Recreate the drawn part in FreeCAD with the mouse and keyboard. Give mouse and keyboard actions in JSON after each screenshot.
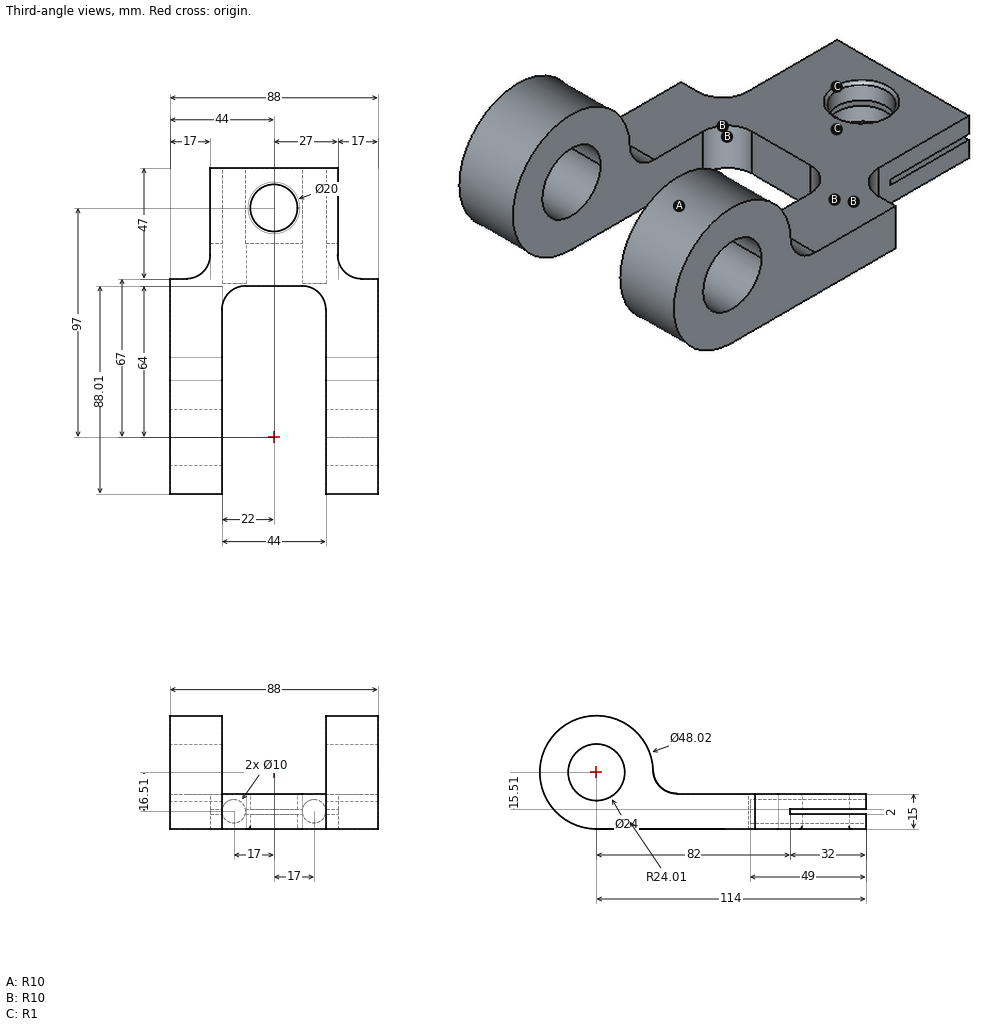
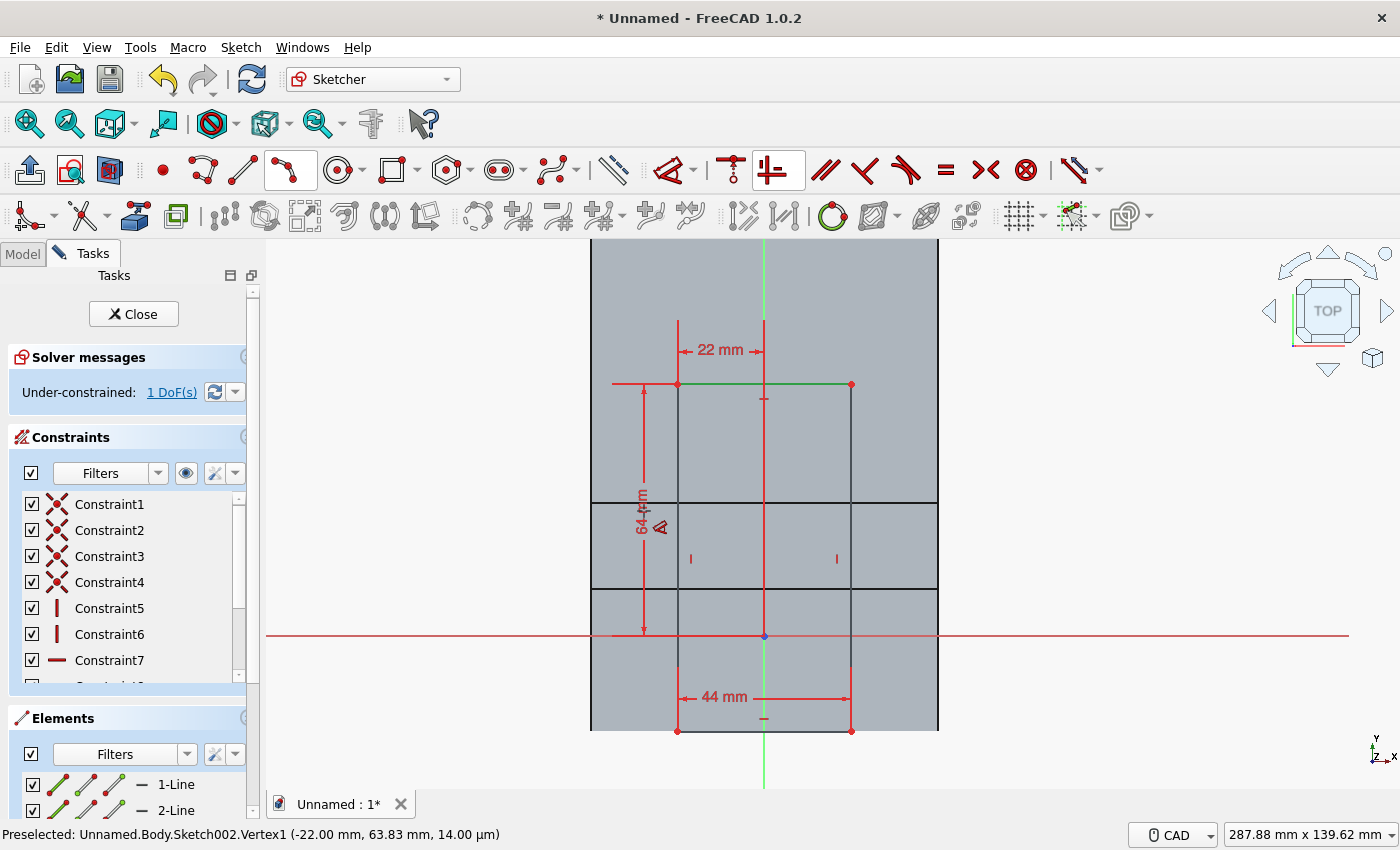
{"action": "left_click", "coordinate": [678, 489]}
{"action": "left_click", "coordinate": [644, 558]}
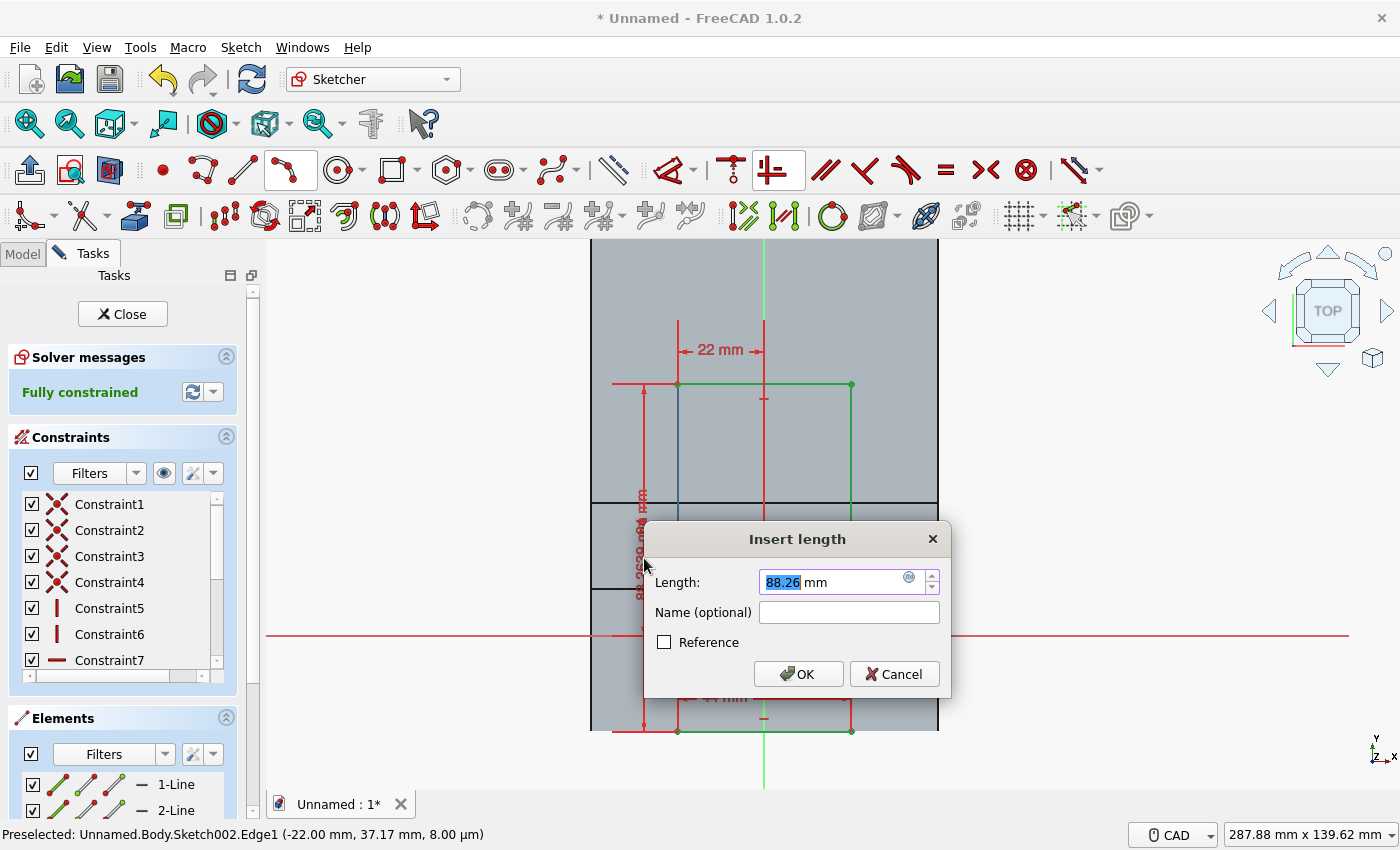
{"action": "type", "text": "88.01"}
{"action": "key", "text": "Return"}
{"action": "key", "text": "Escape"}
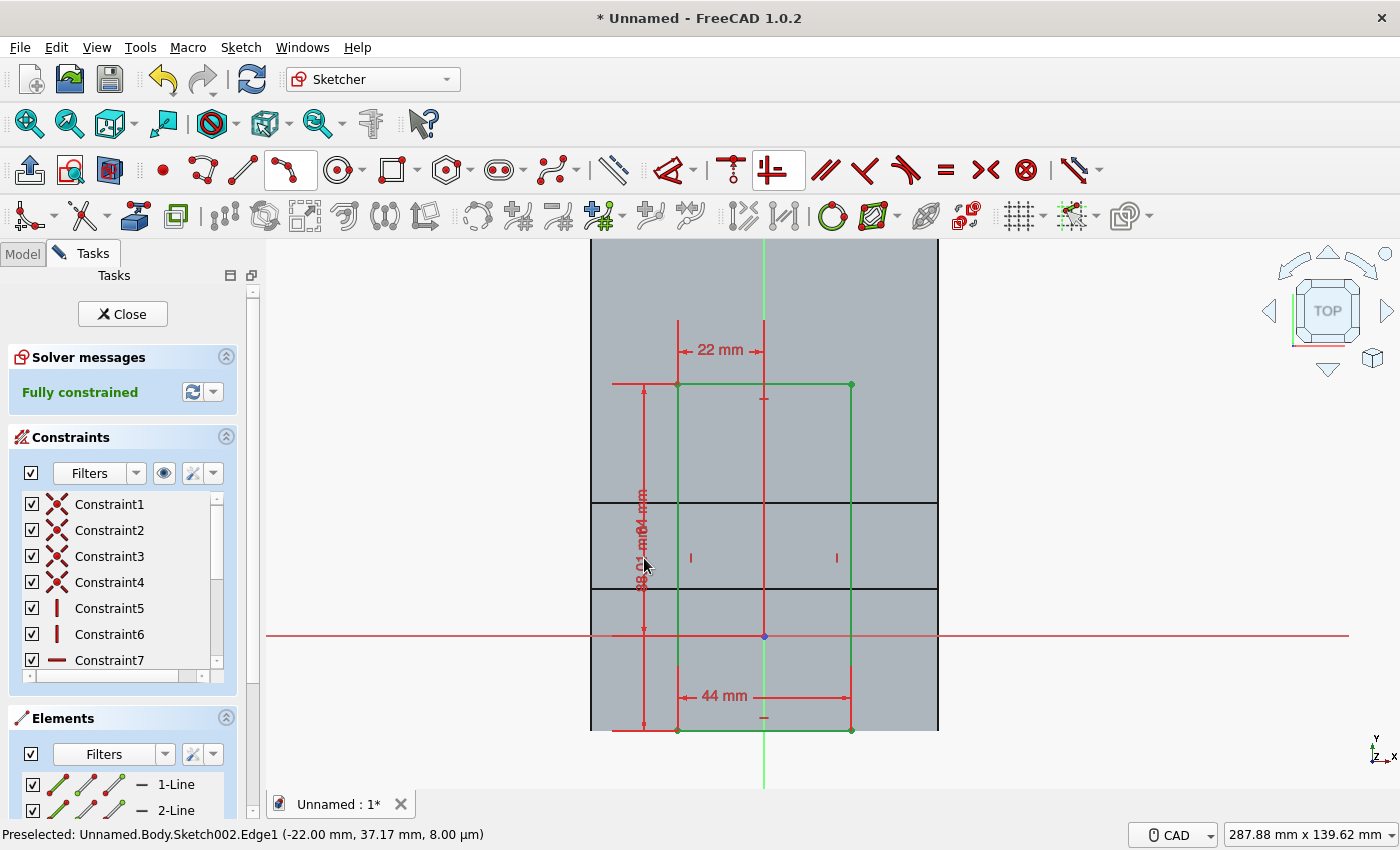
{"action": "left_click", "coordinate": [123, 314]}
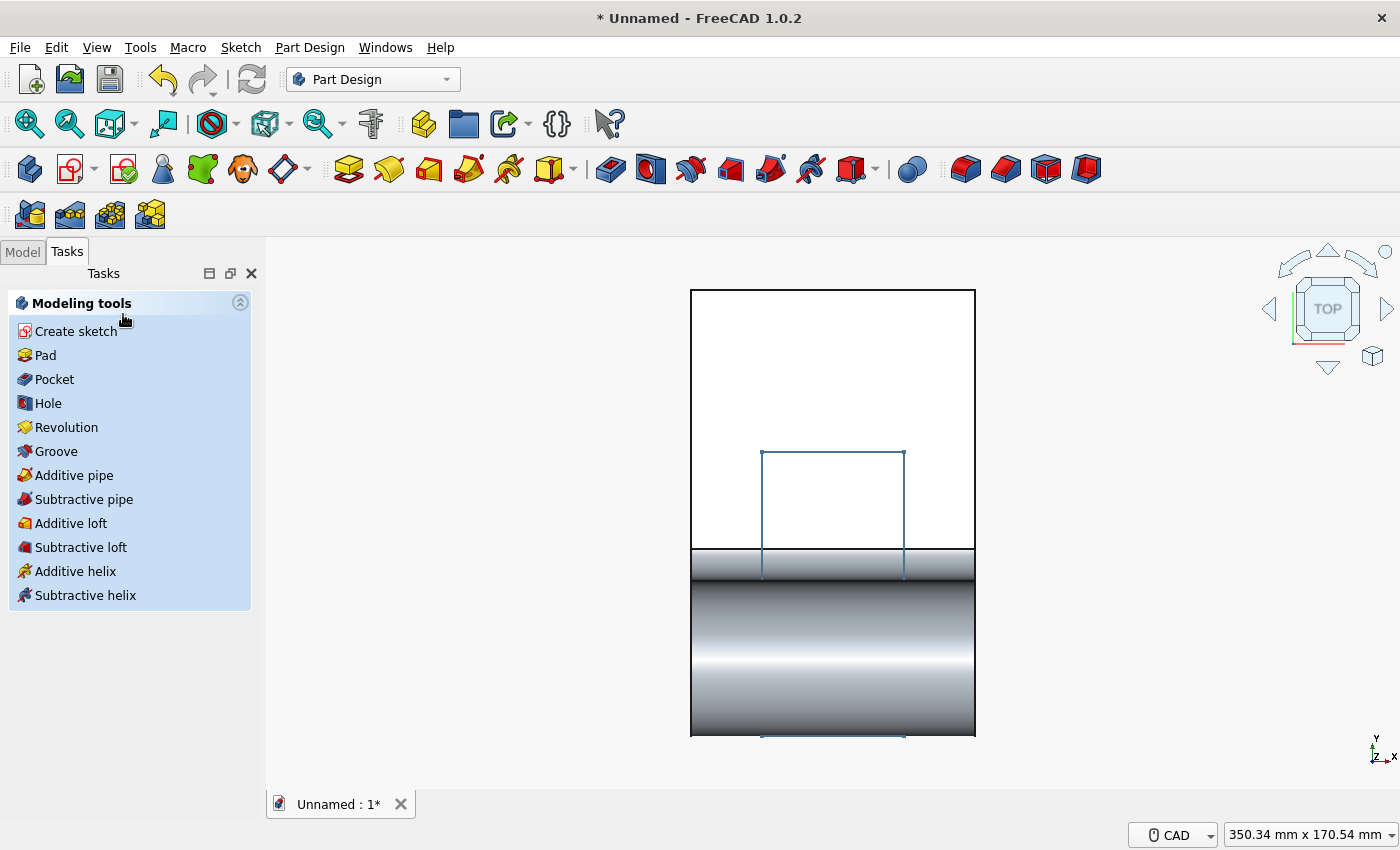
{"action": "left_click", "coordinate": [612, 170]}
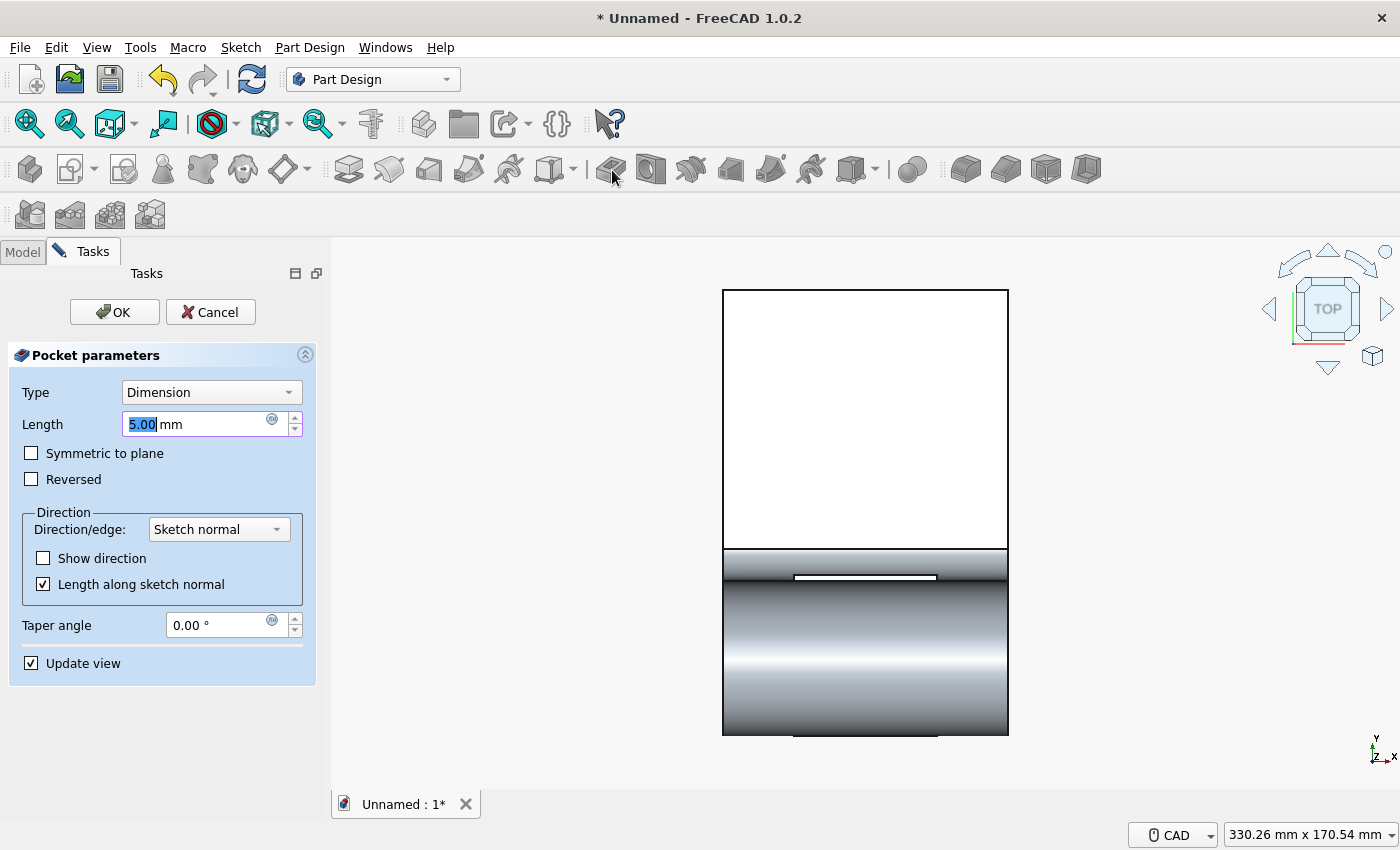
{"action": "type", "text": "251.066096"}
{"action": "key", "text": "Tab"}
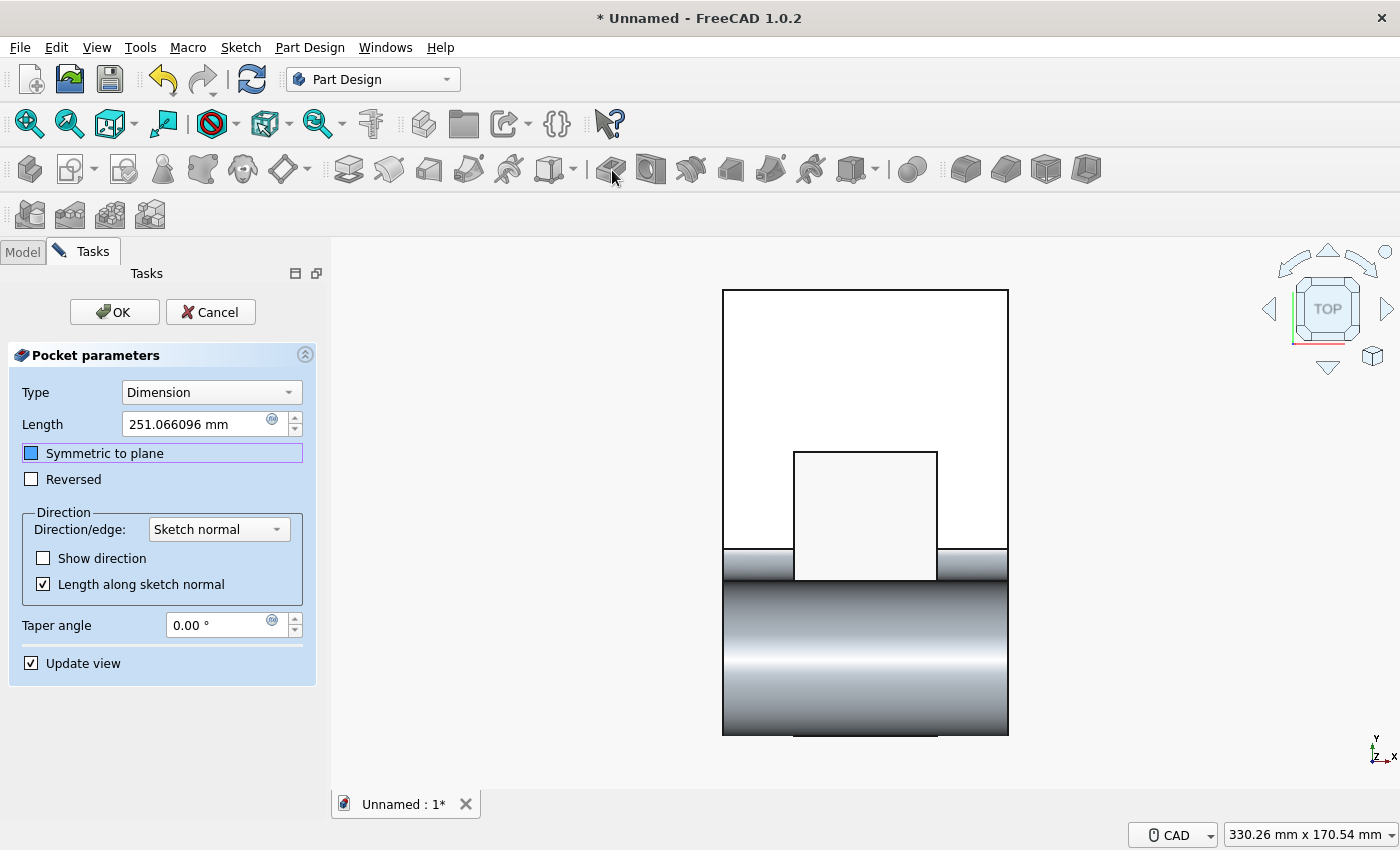
{"action": "left_click", "coordinate": [30, 453]}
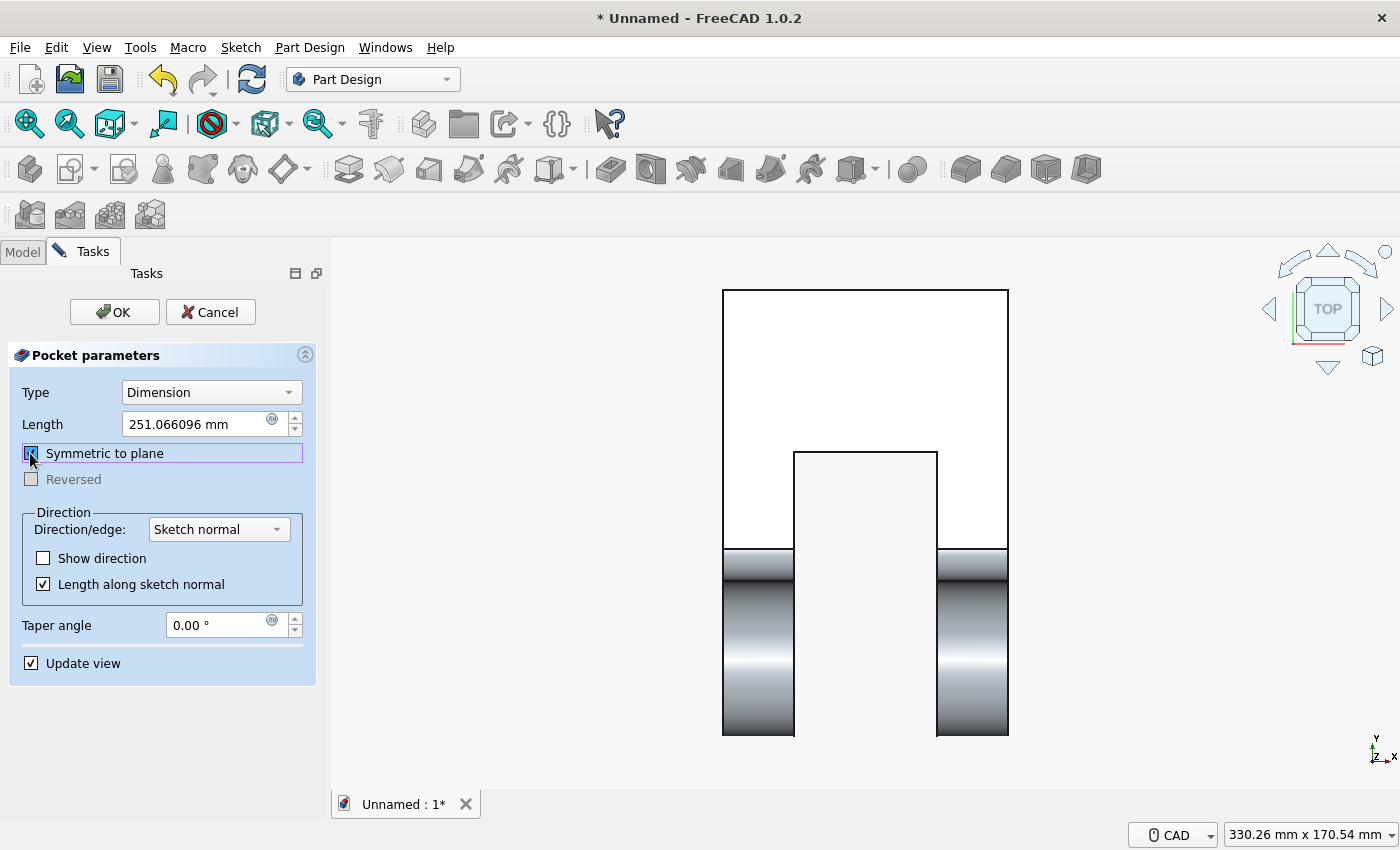
{"action": "left_click", "coordinate": [115, 312]}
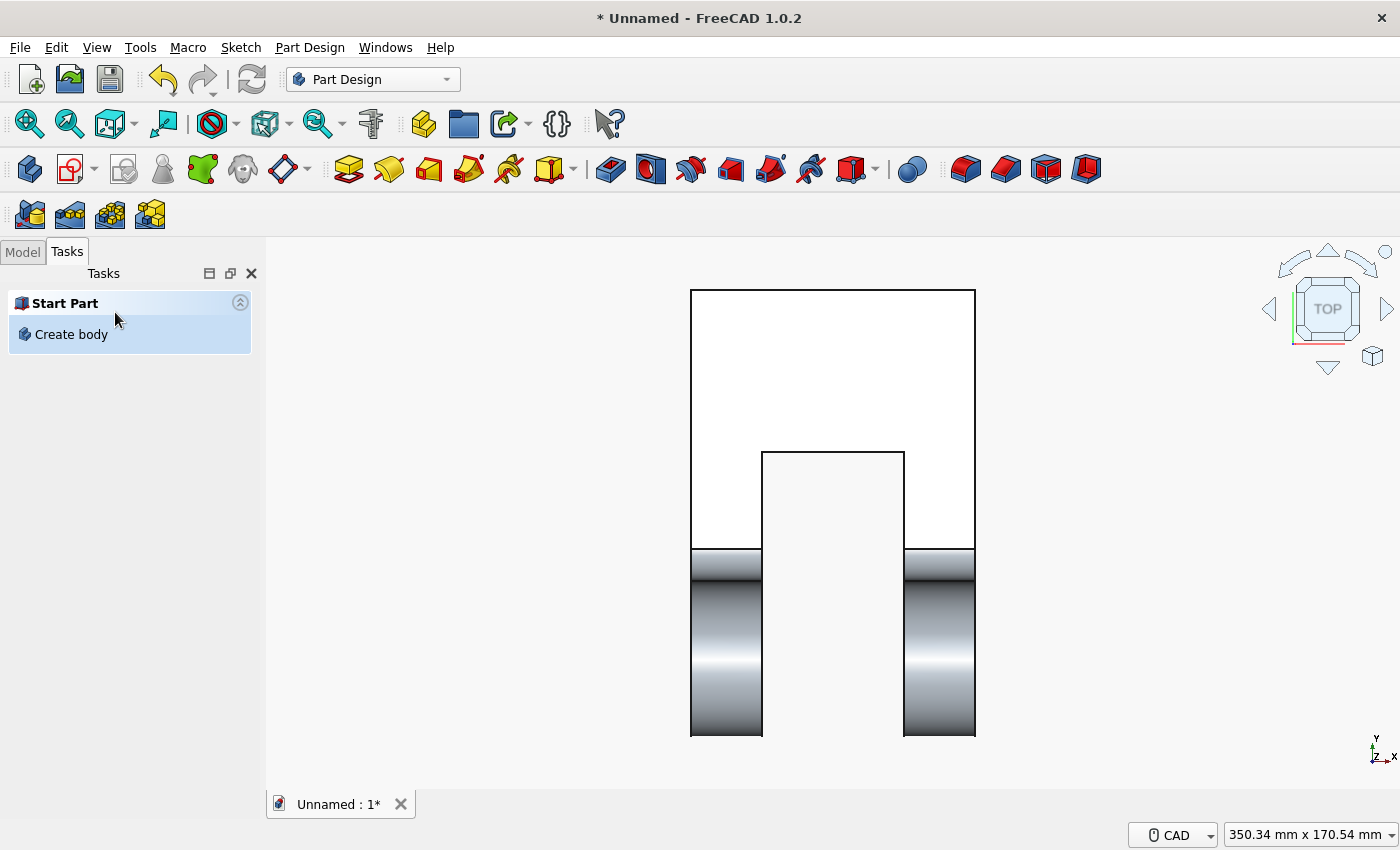
{"action": "left_click", "coordinate": [70, 170]}